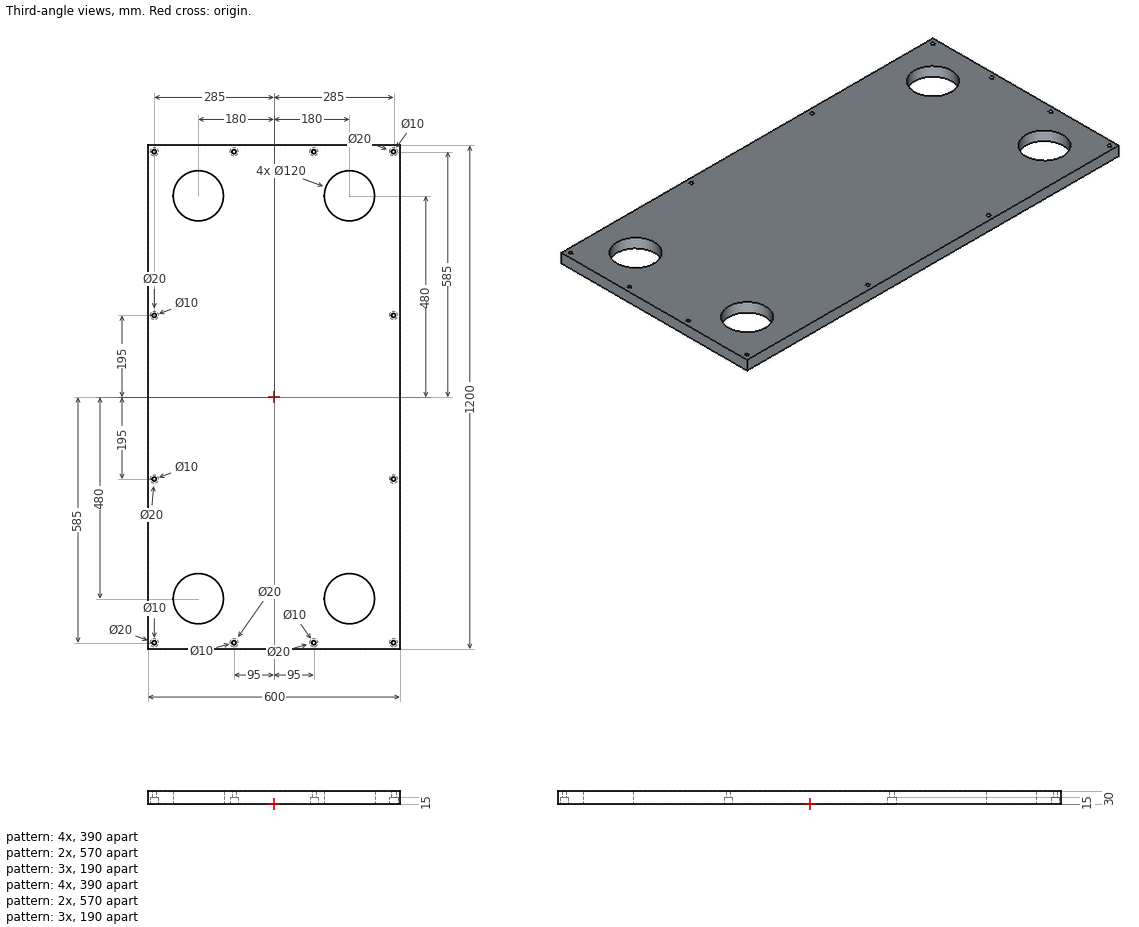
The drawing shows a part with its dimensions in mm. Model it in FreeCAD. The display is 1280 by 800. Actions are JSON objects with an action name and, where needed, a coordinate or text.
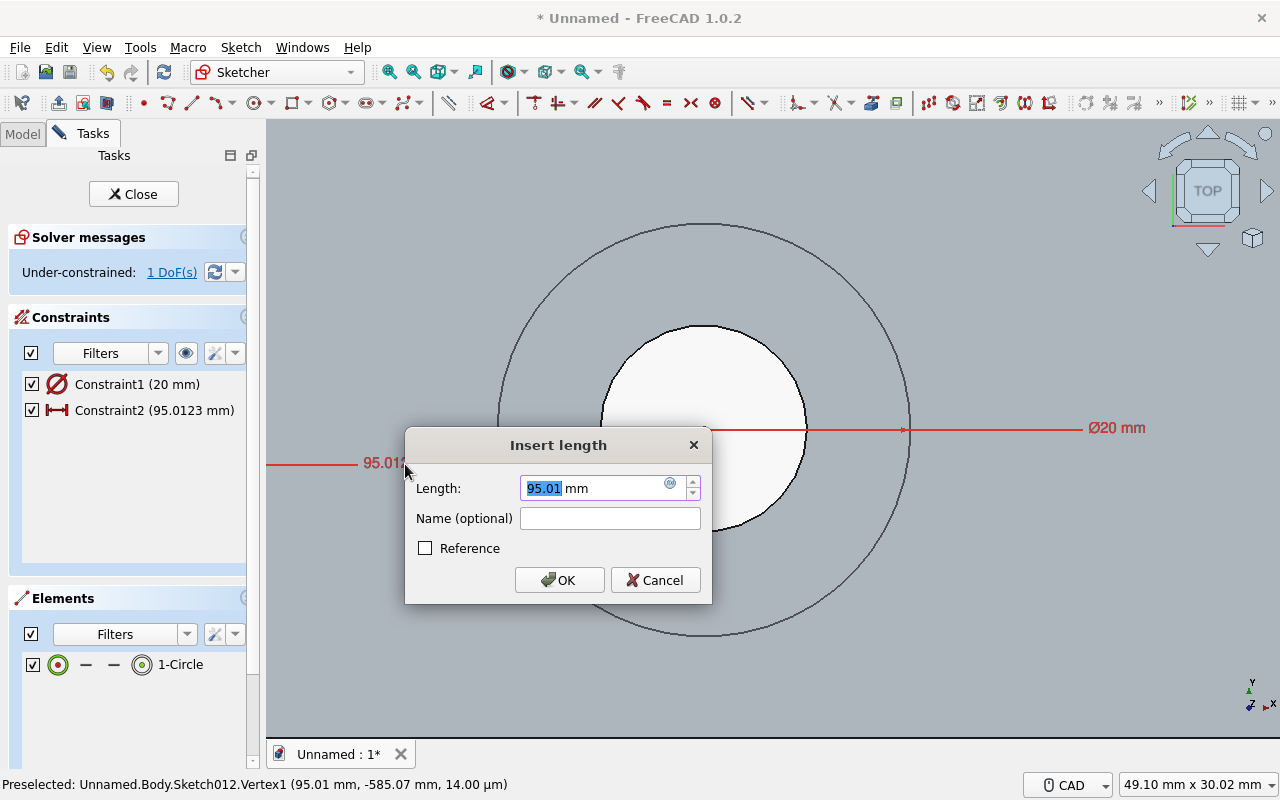
{"action": "type", "text": "95"}
{"action": "key", "text": "Return"}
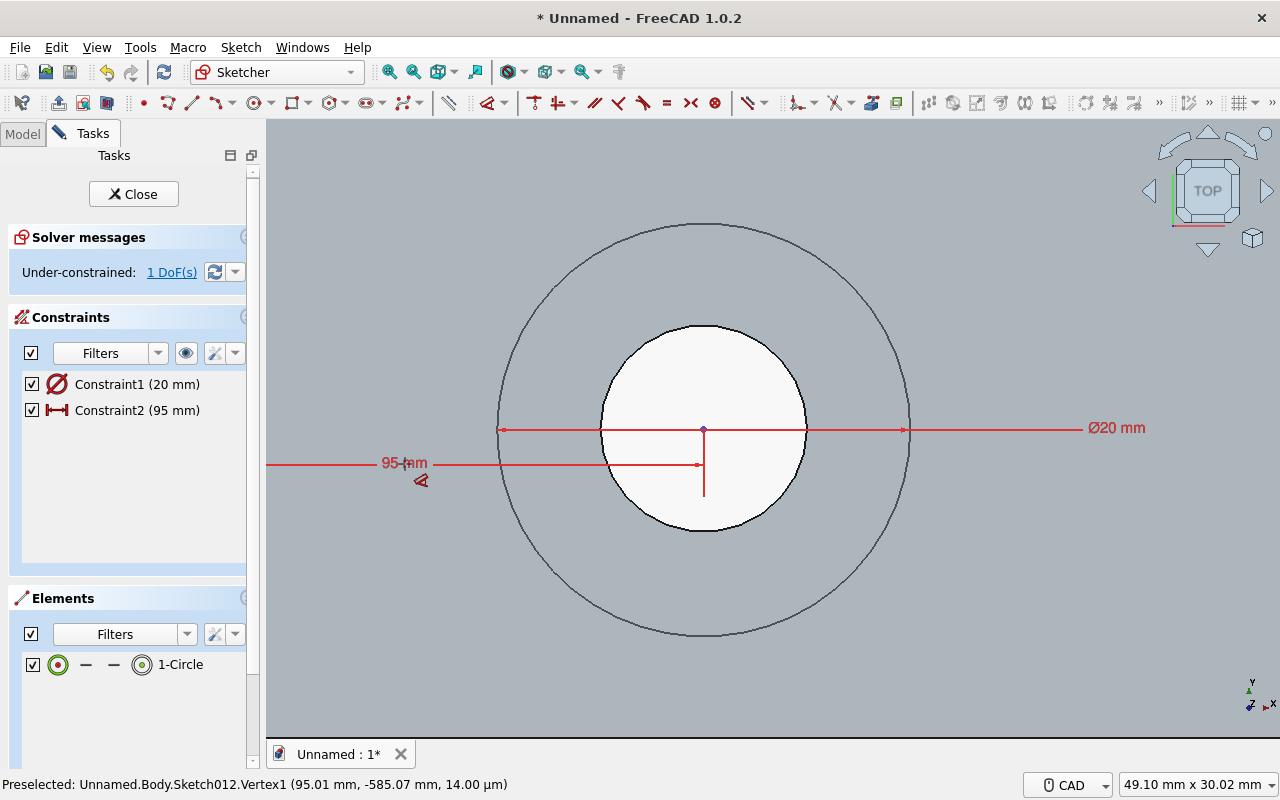
{"action": "left_click", "coordinate": [704, 430]}
{"action": "left_click", "coordinate": [738, 288]}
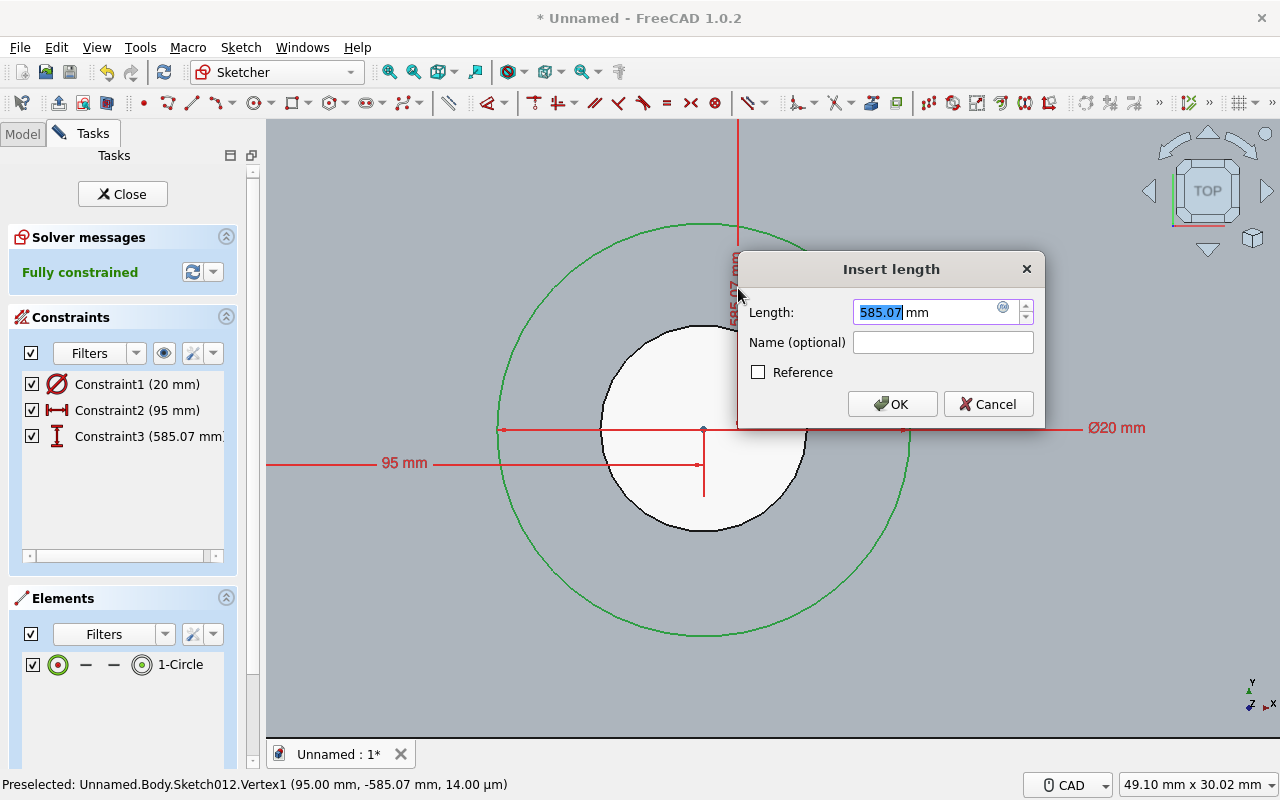
{"action": "type", "text": "585"}
{"action": "key", "text": "Return"}
{"action": "key", "text": "Escape"}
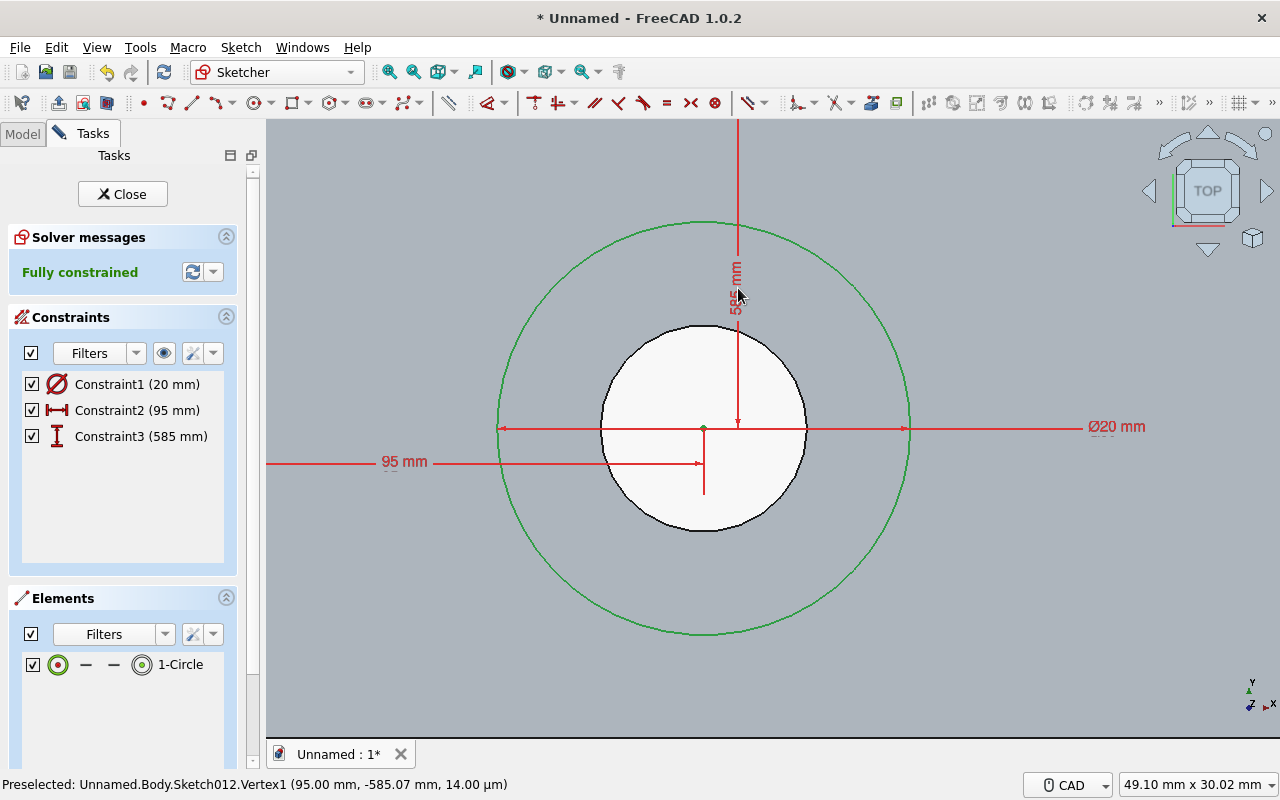
{"action": "left_click", "coordinate": [123, 194]}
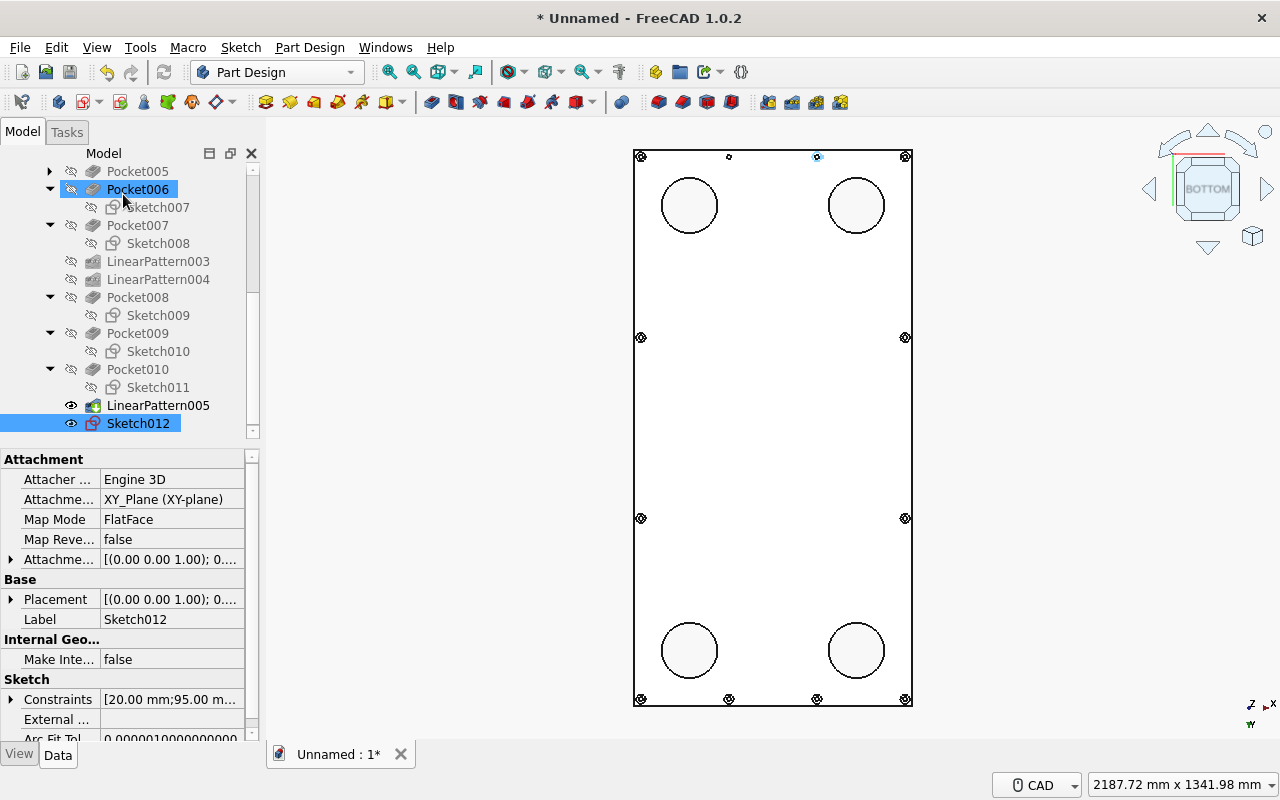
{"action": "left_click", "coordinate": [432, 102]}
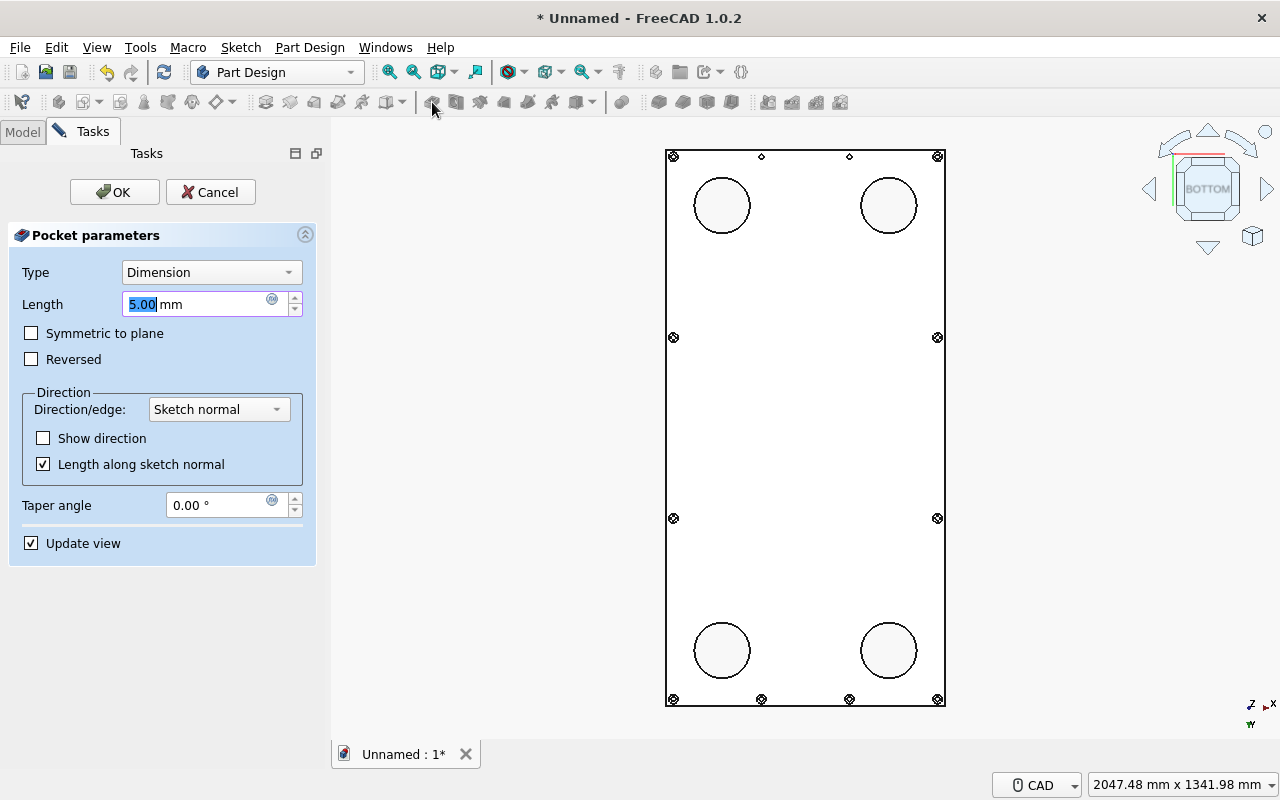
{"action": "type", "text": "15"}
{"action": "key", "text": "Tab"}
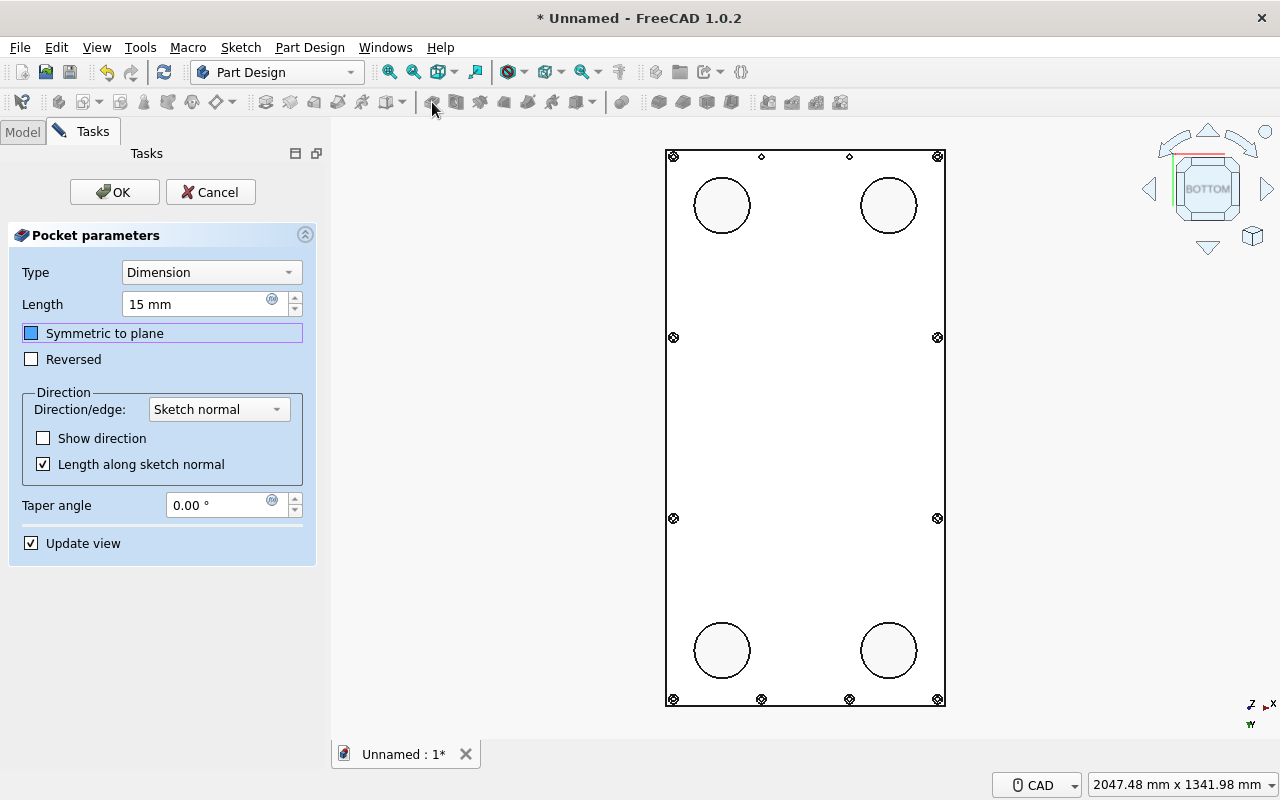
{"action": "left_click", "coordinate": [30, 359]}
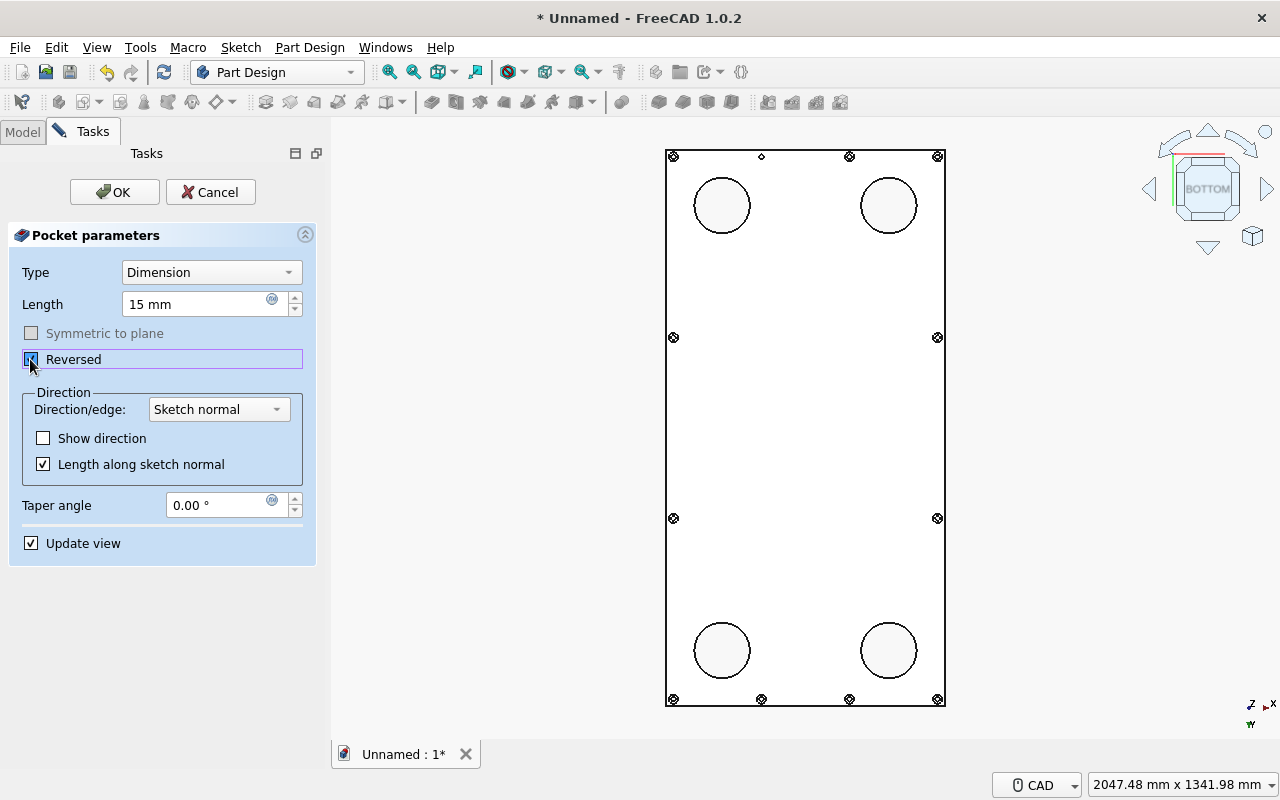
{"action": "left_click", "coordinate": [115, 192]}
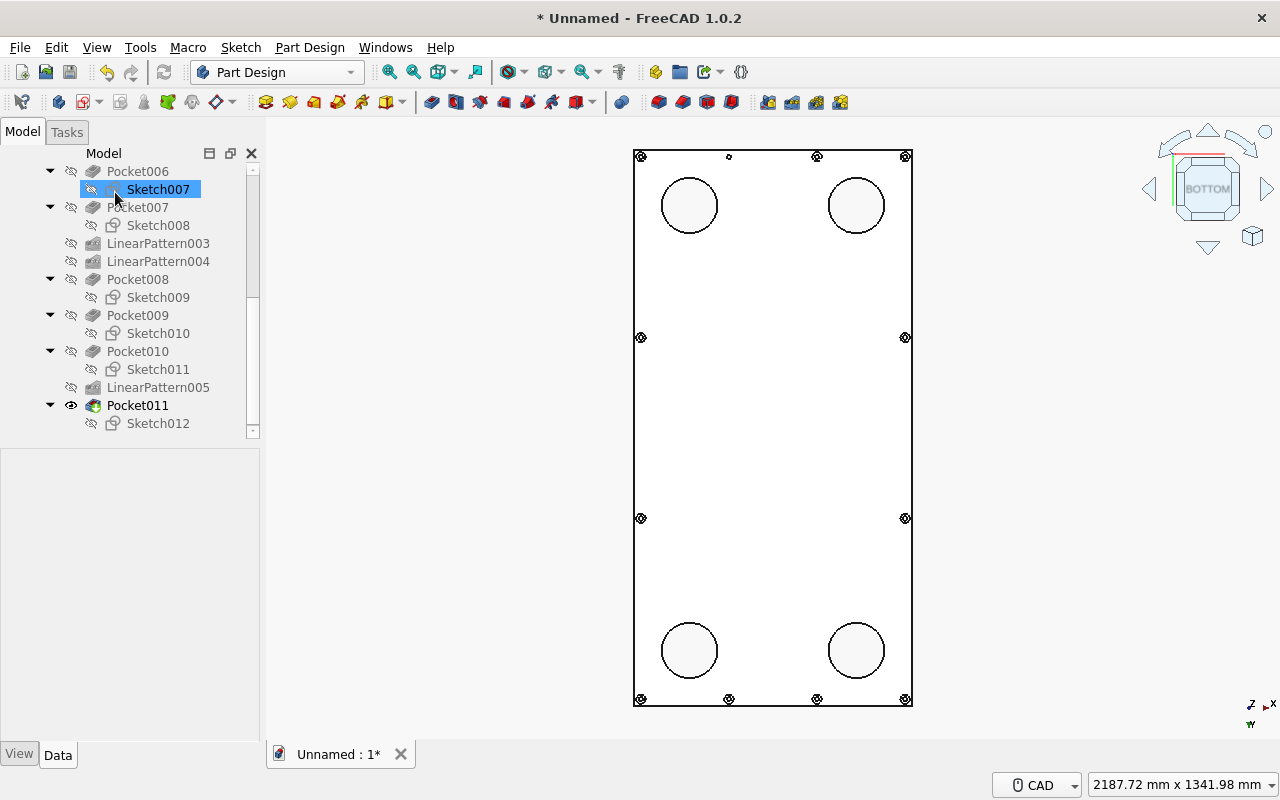
{"action": "left_click", "coordinate": [84, 102]}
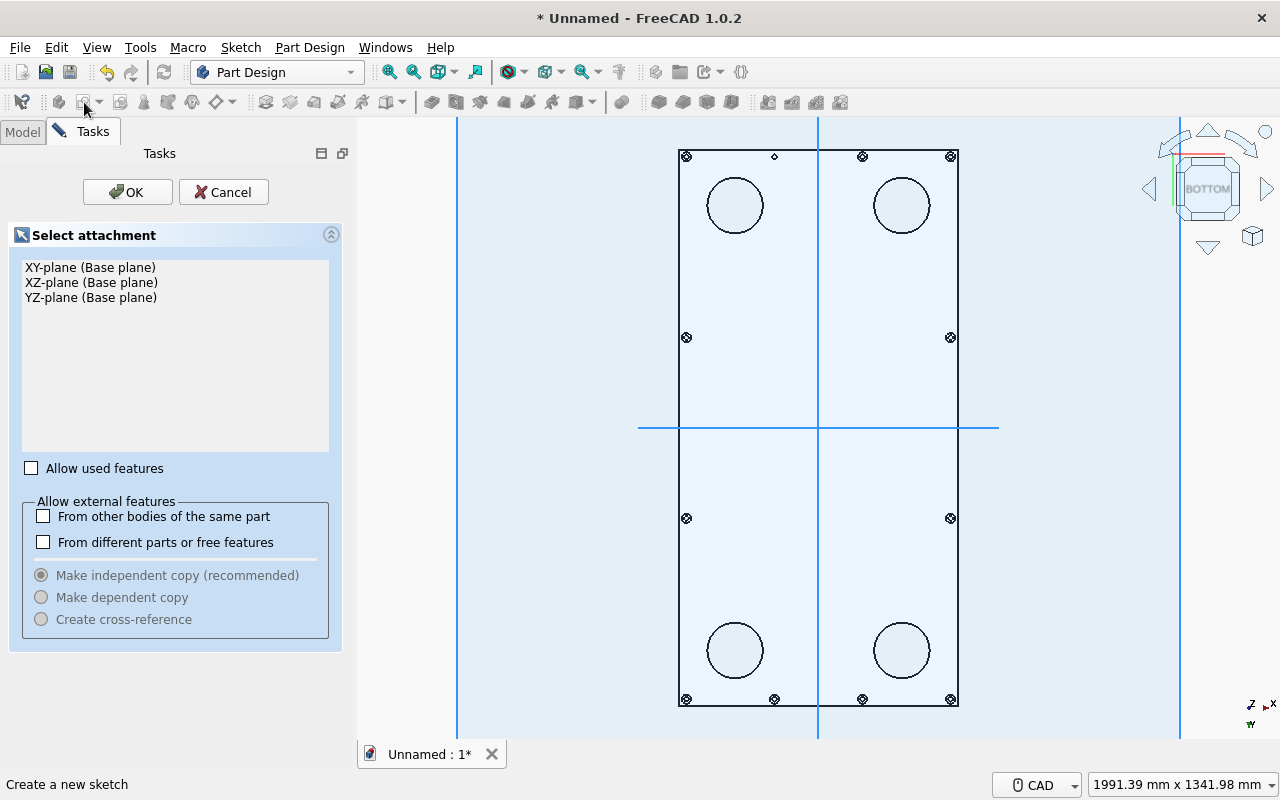
{"action": "left_click", "coordinate": [82, 268]}